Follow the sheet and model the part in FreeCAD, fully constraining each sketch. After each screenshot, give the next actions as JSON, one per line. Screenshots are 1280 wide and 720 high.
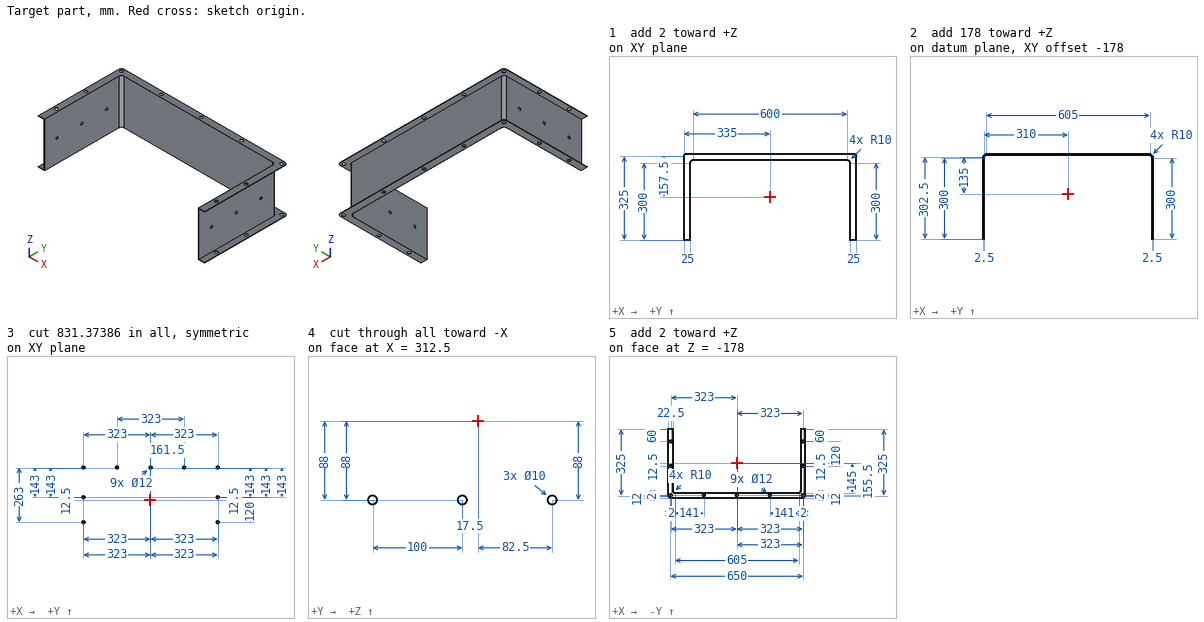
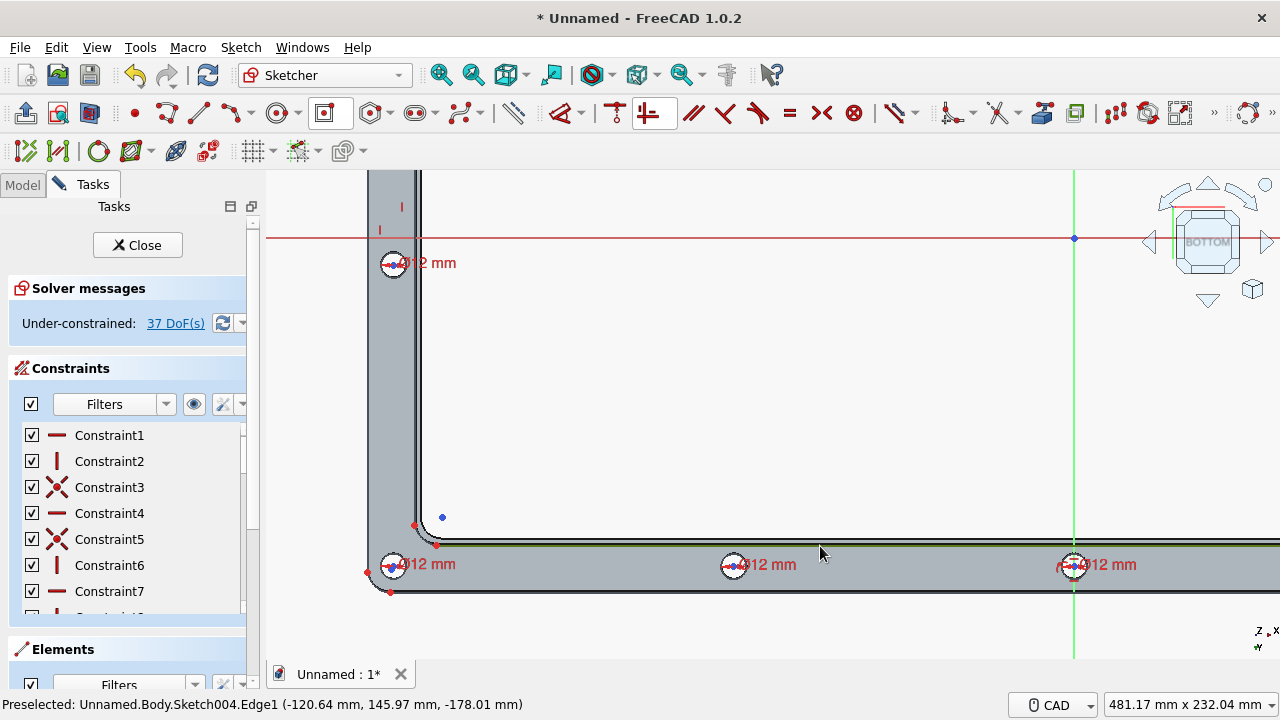
{"action": "scroll", "coordinate": [419, 534], "scroll_direction": "up", "scroll_amount": 2}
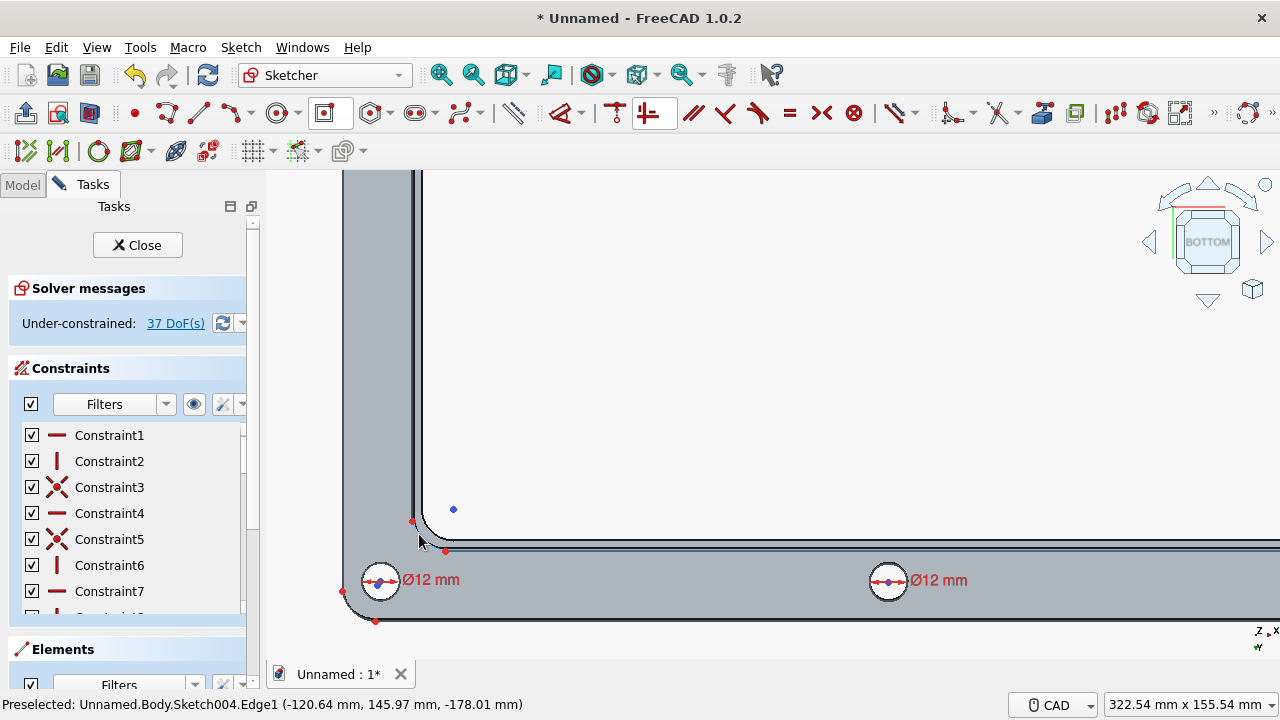
{"action": "left_click", "coordinate": [419, 534]}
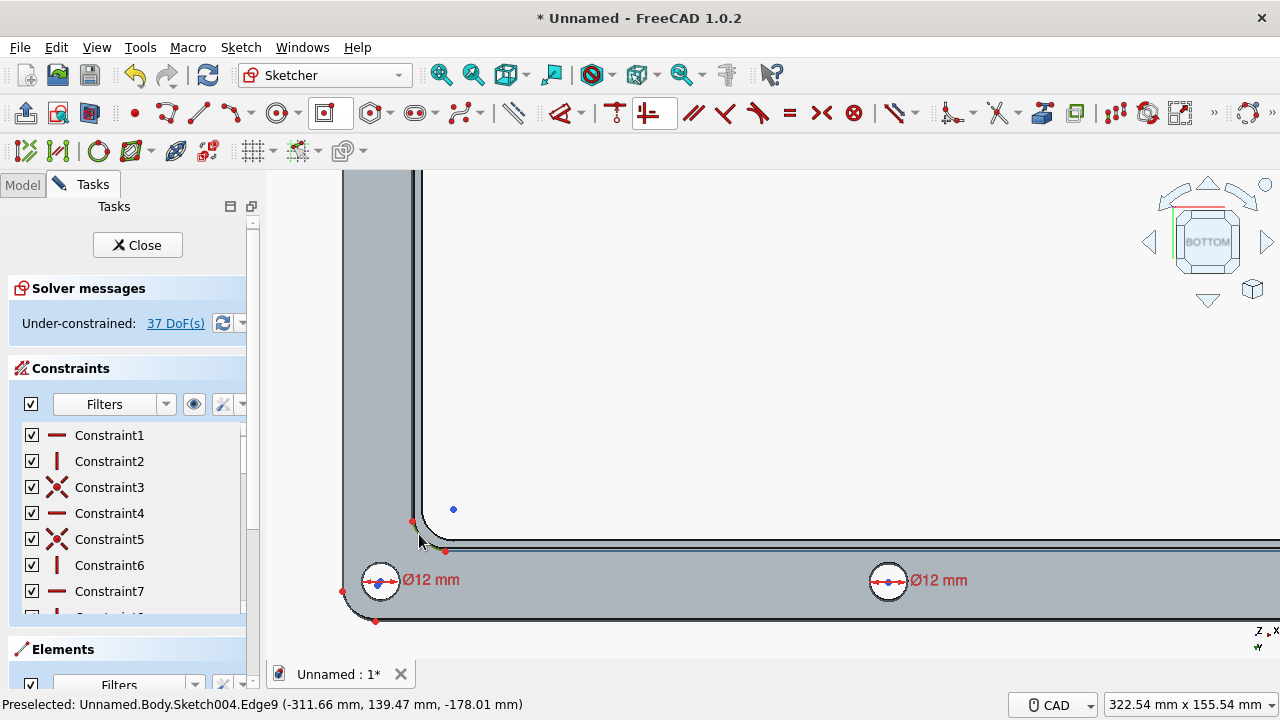
{"action": "key", "text": "t"}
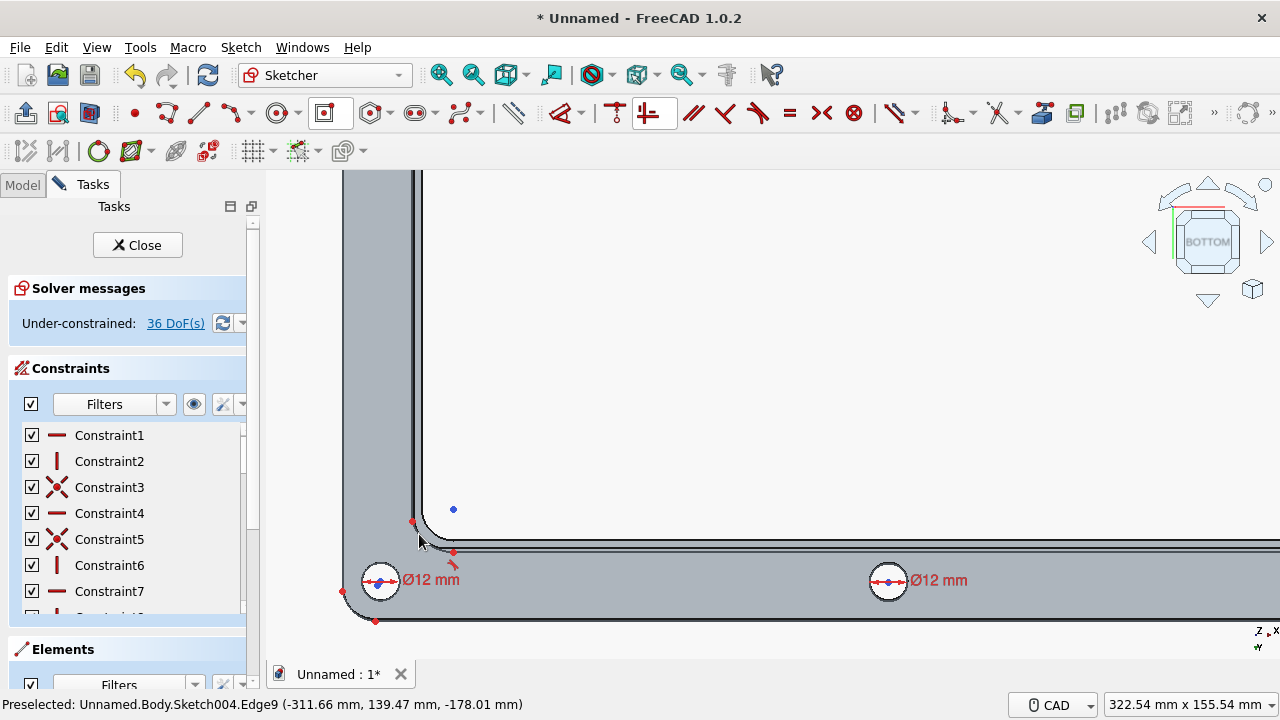
{"action": "left_click", "coordinate": [1022, 552]}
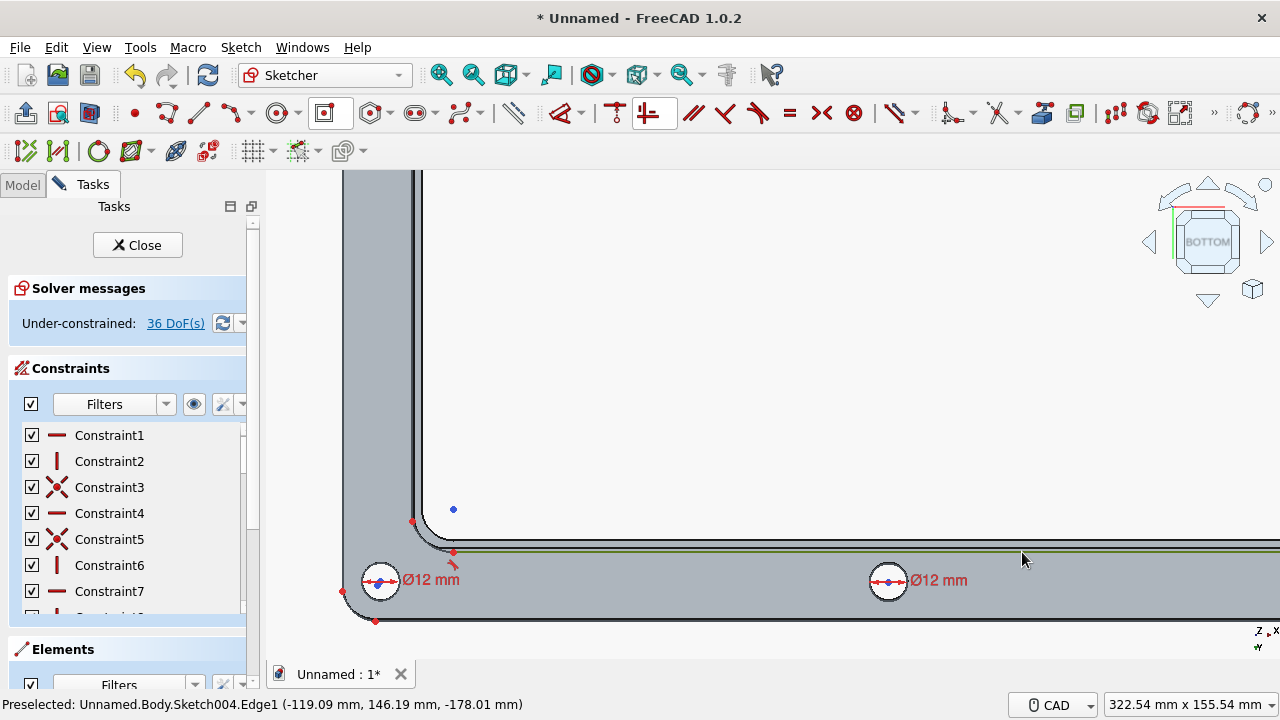
{"action": "scroll", "coordinate": [406, 553], "scroll_direction": "down", "scroll_amount": 6}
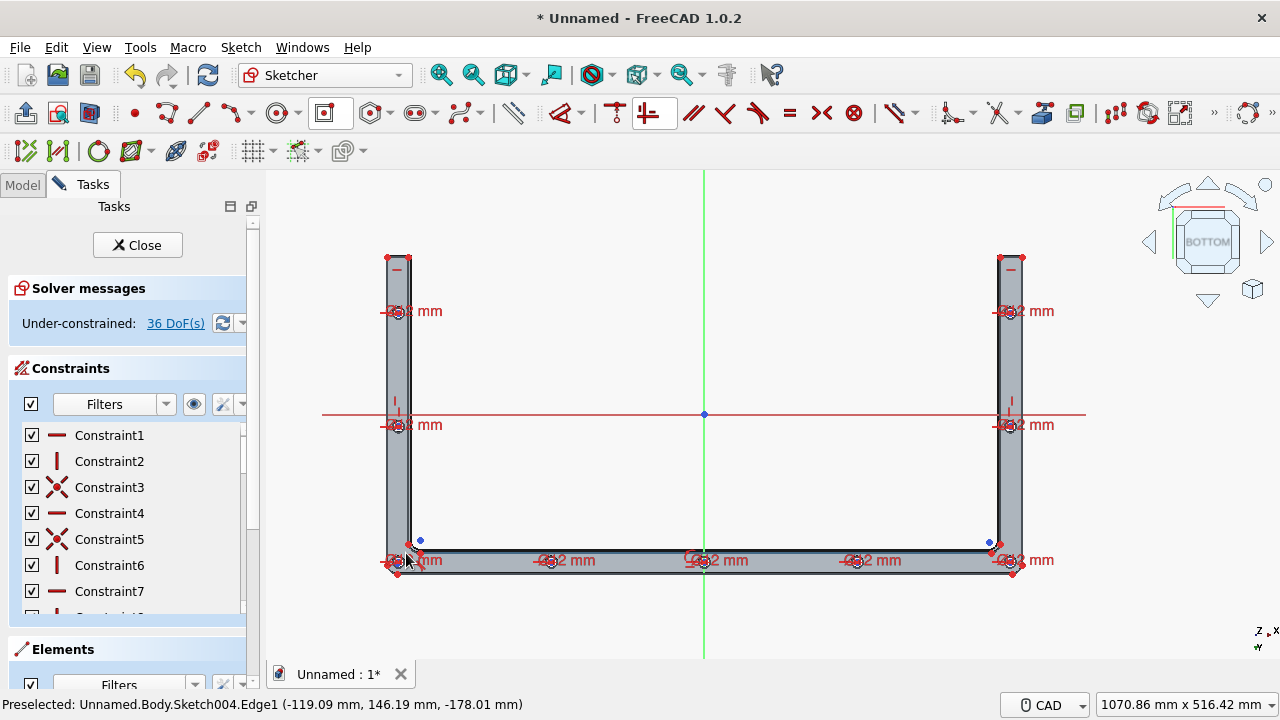
{"action": "scroll", "coordinate": [995, 552], "scroll_direction": "up", "scroll_amount": 6}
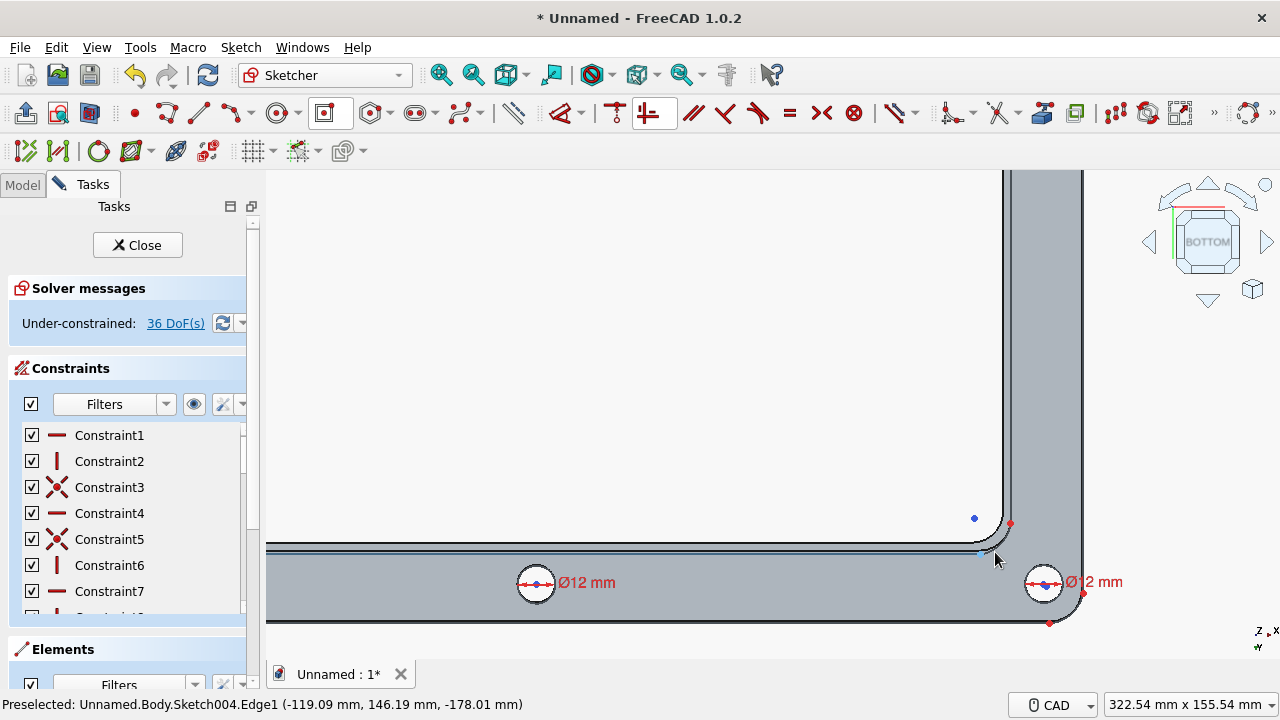
{"action": "left_click", "coordinate": [993, 550]}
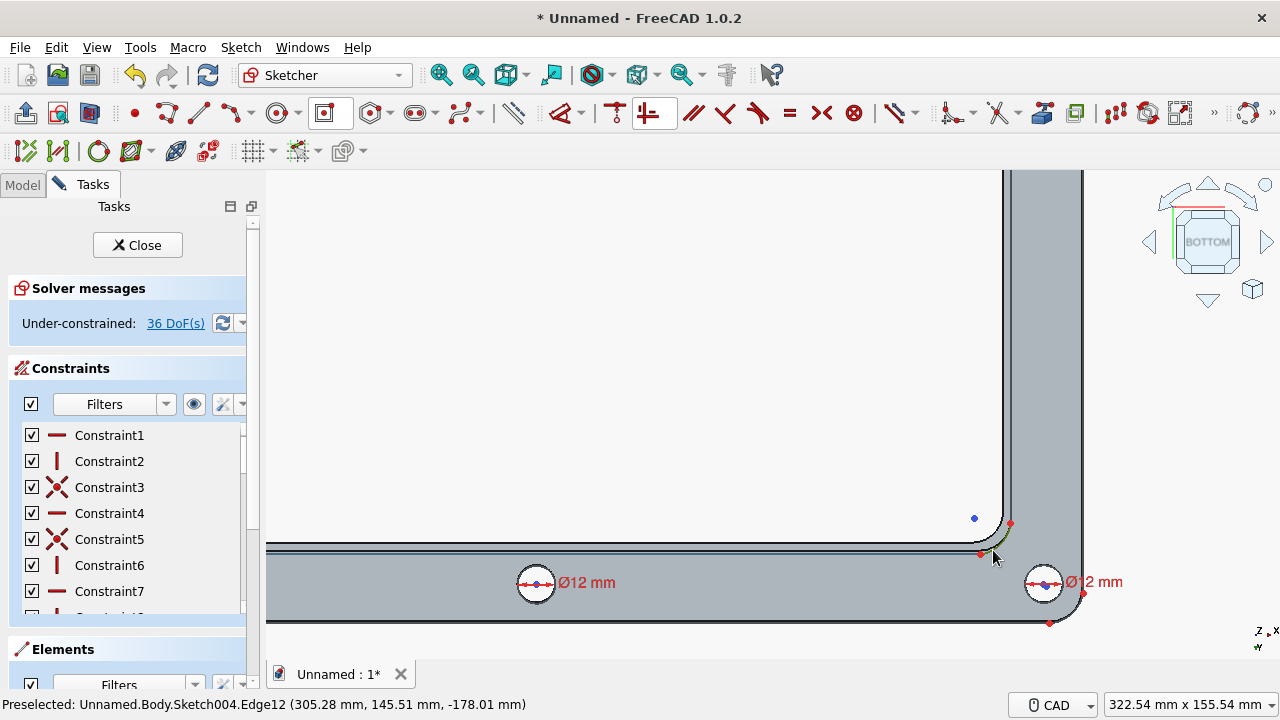
{"action": "left_click", "coordinate": [758, 114]}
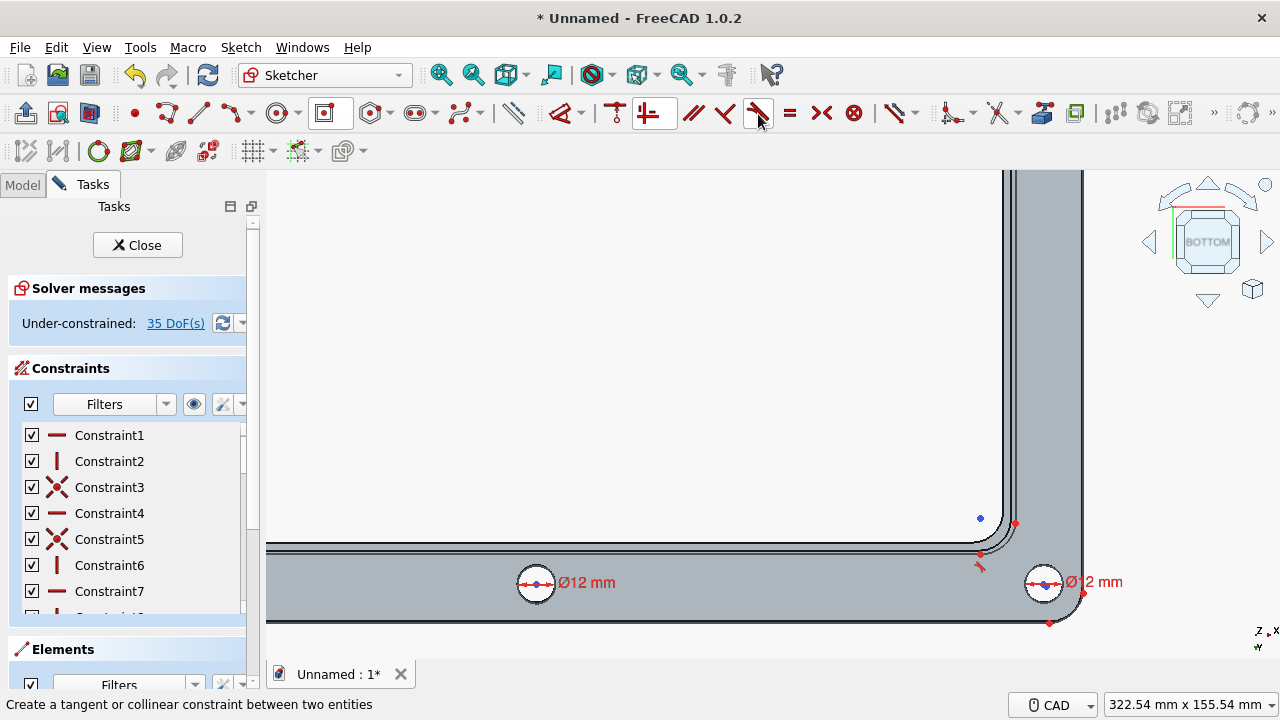
{"action": "scroll", "coordinate": [996, 552], "scroll_direction": "down", "scroll_amount": 6}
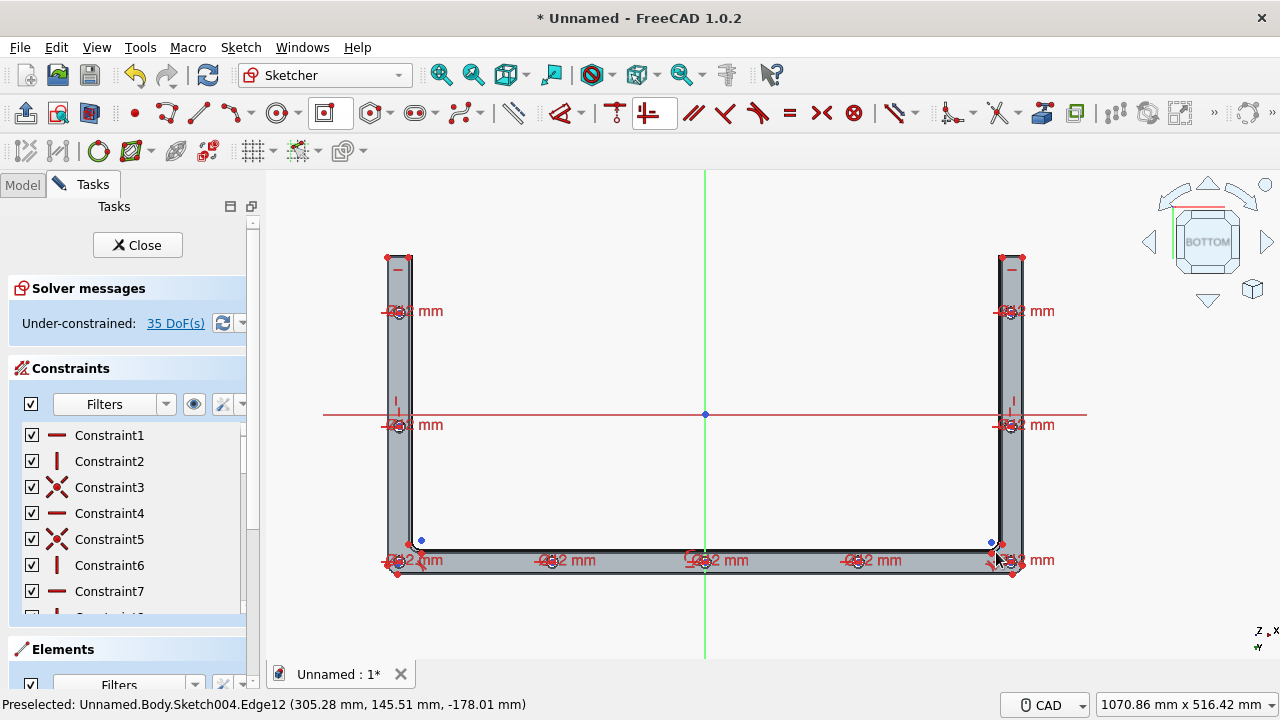
{"action": "left_click", "coordinate": [409, 458]}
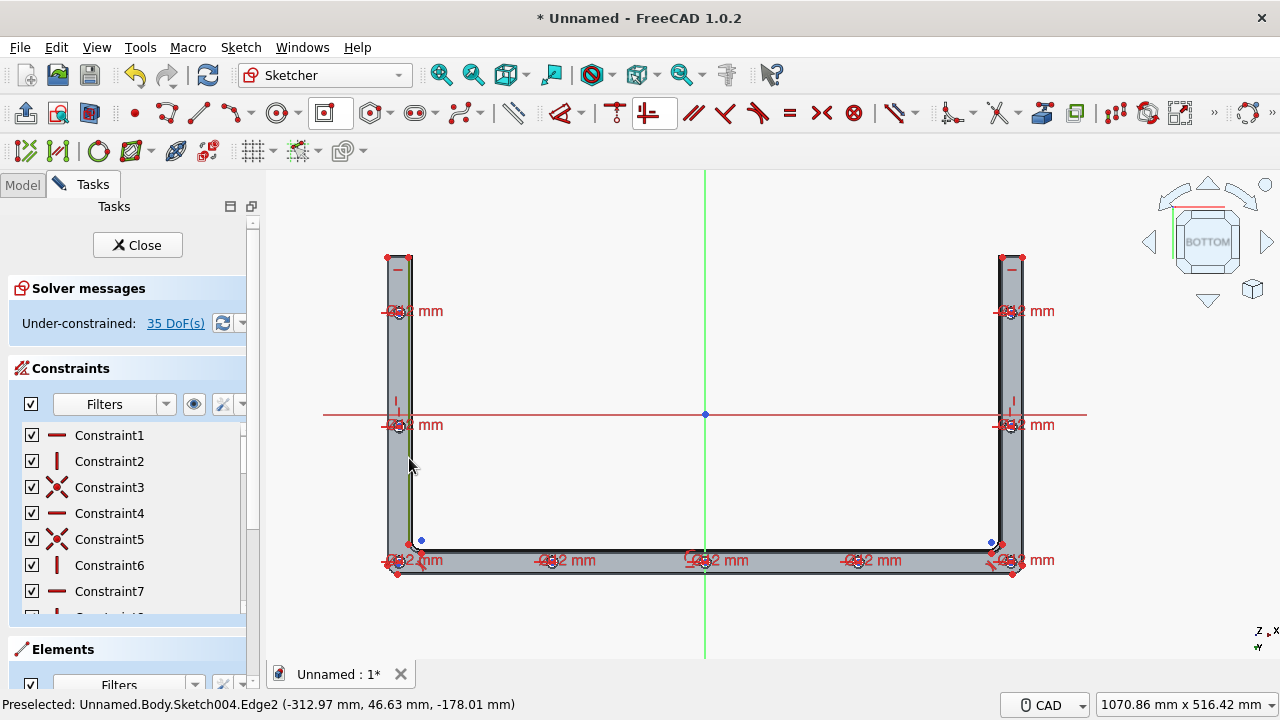
{"action": "scroll", "coordinate": [413, 551], "scroll_direction": "up", "scroll_amount": 3}